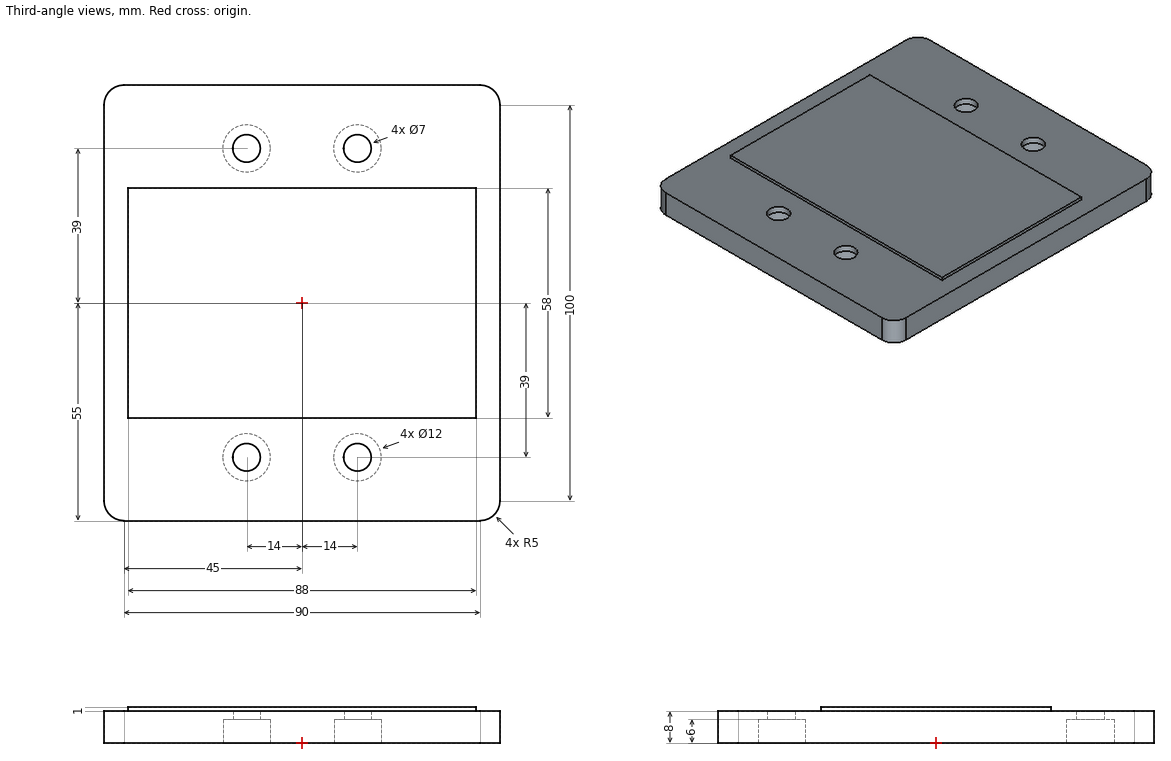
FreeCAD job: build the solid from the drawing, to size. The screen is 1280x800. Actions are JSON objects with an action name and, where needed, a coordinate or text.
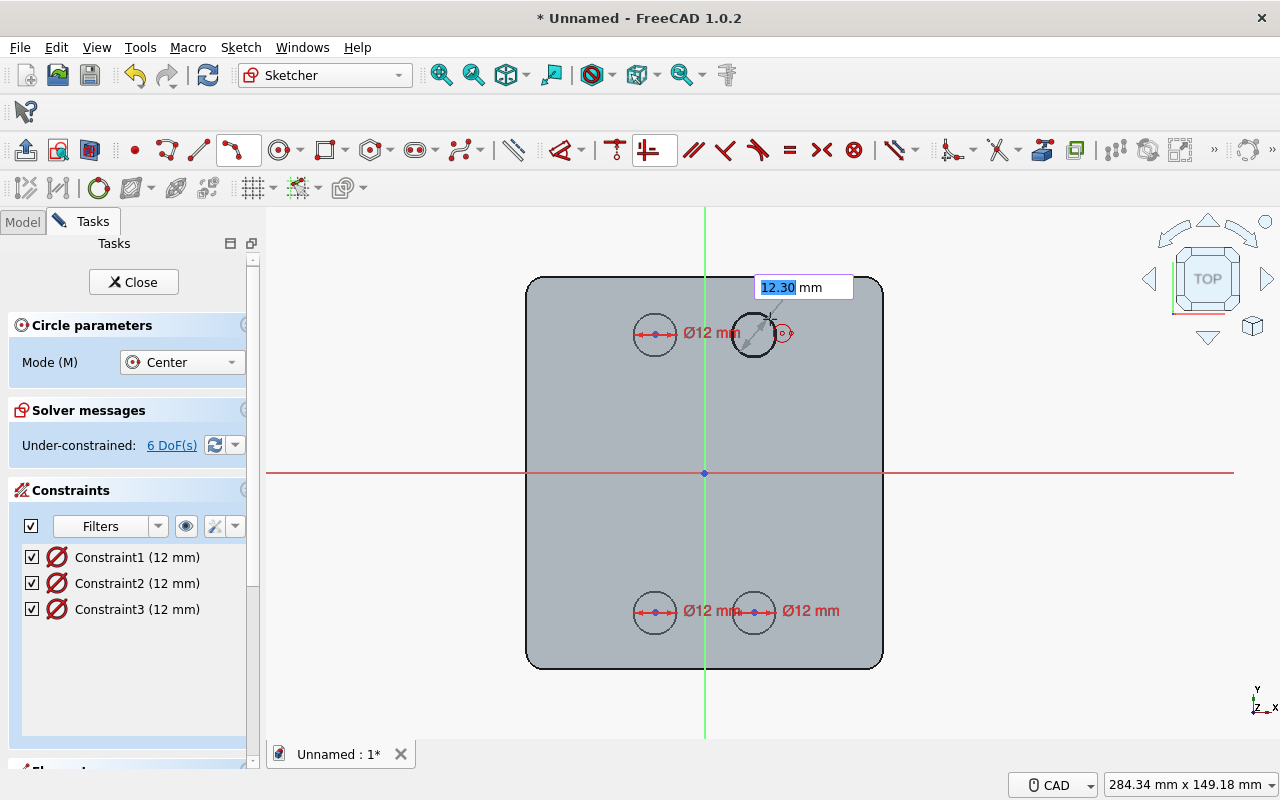
{"action": "type", "text": "12"}
{"action": "key", "text": "Return"}
{"action": "key", "text": "Escape"}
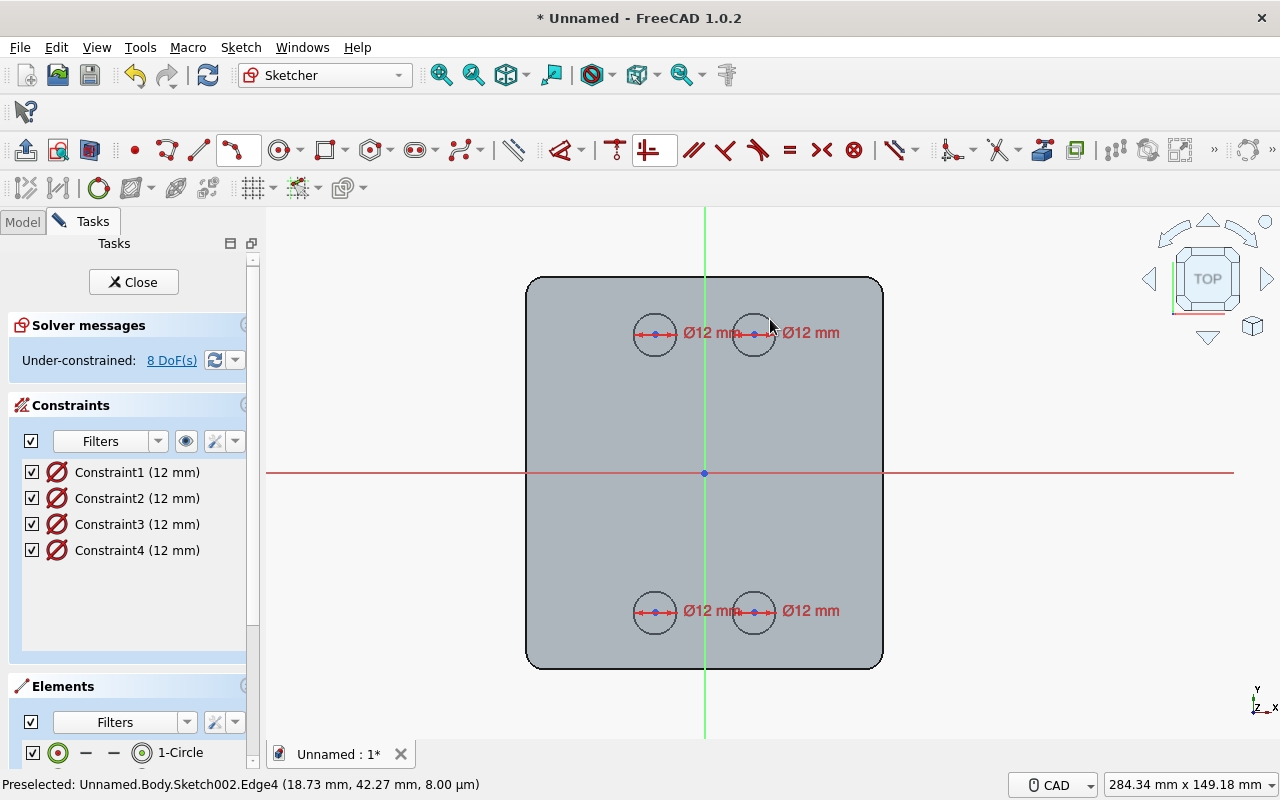
{"action": "left_click", "coordinate": [754, 613]}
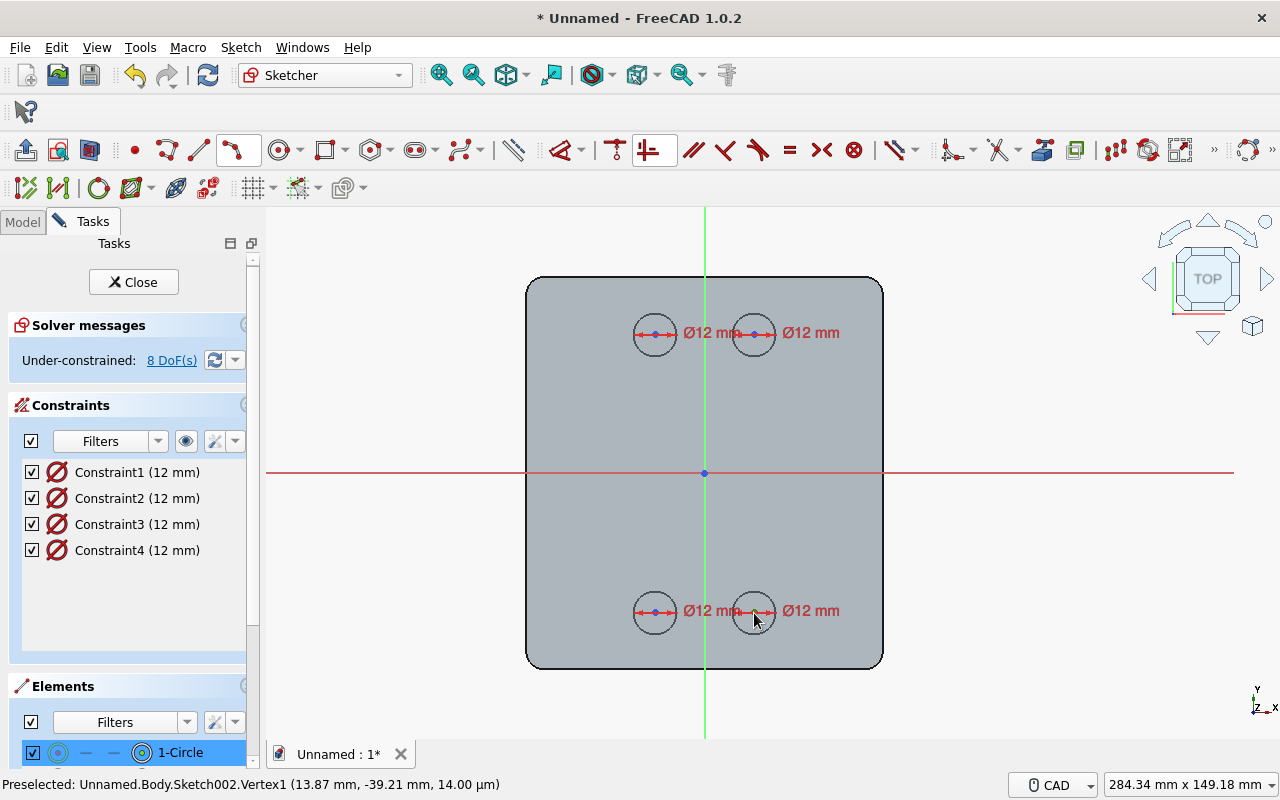
{"action": "left_click", "coordinate": [655, 613]}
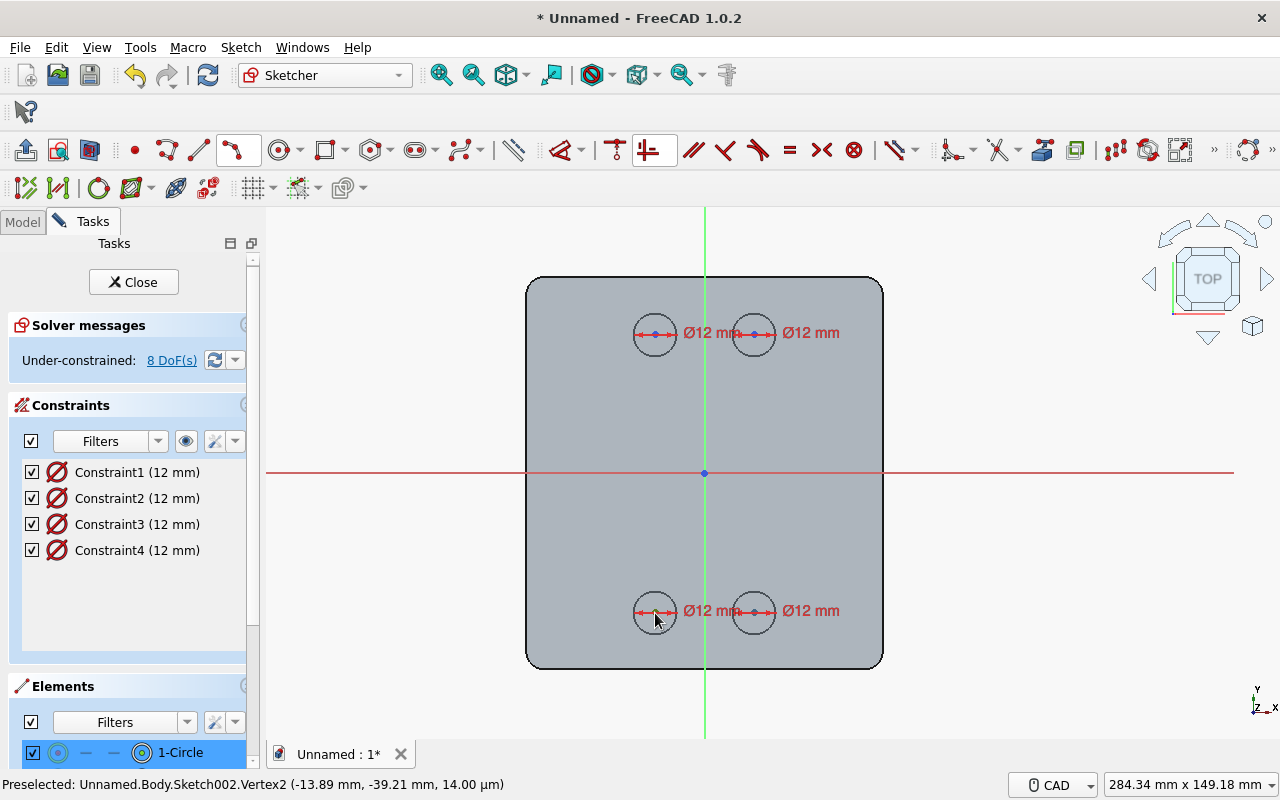
{"action": "key", "text": "h"}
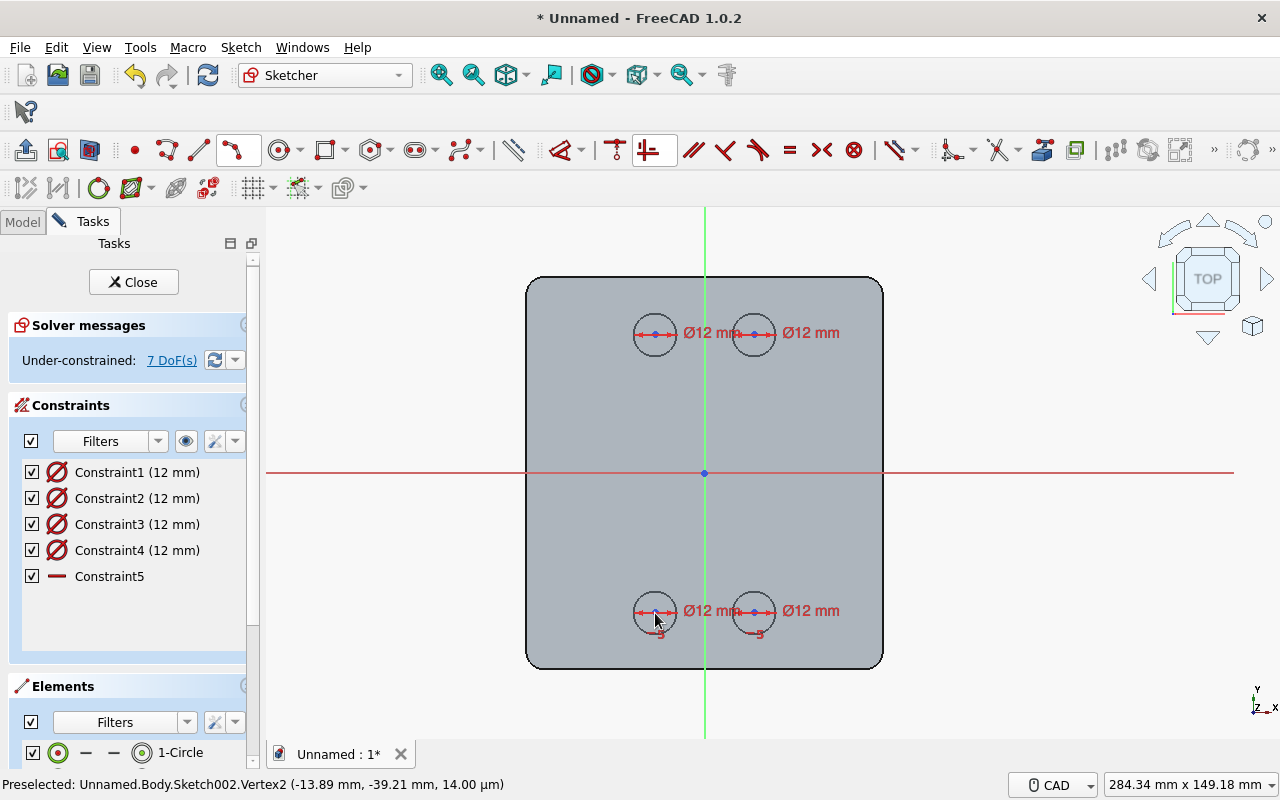
{"action": "left_click", "coordinate": [655, 613]}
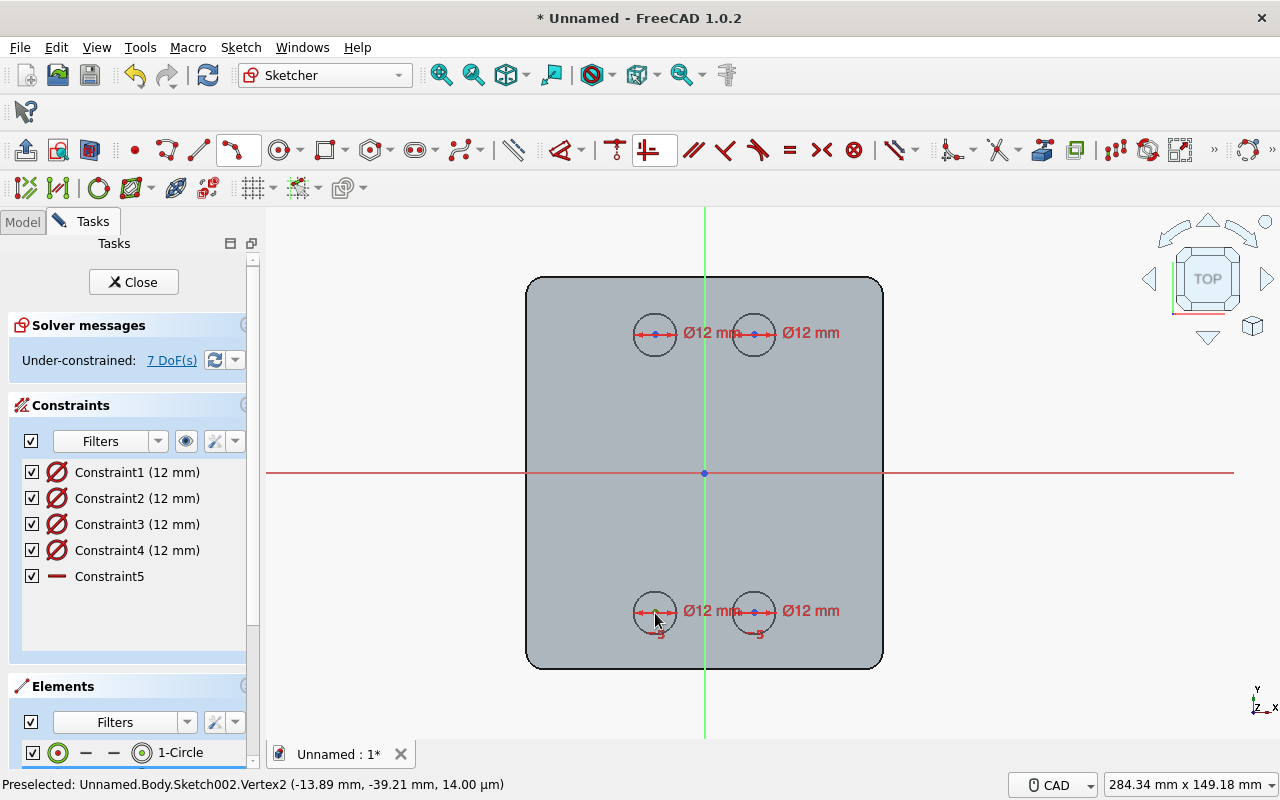
{"action": "left_click", "coordinate": [655, 335]}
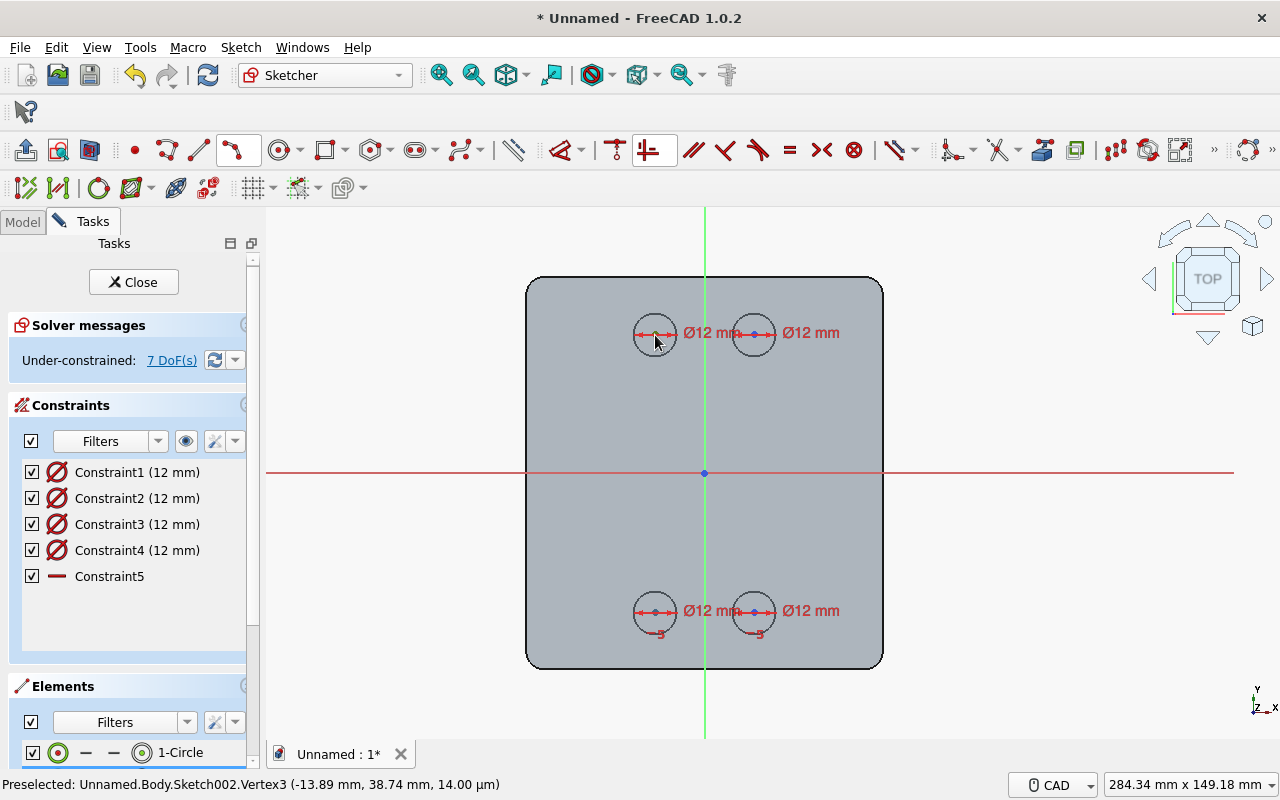
{"action": "key", "text": "v"}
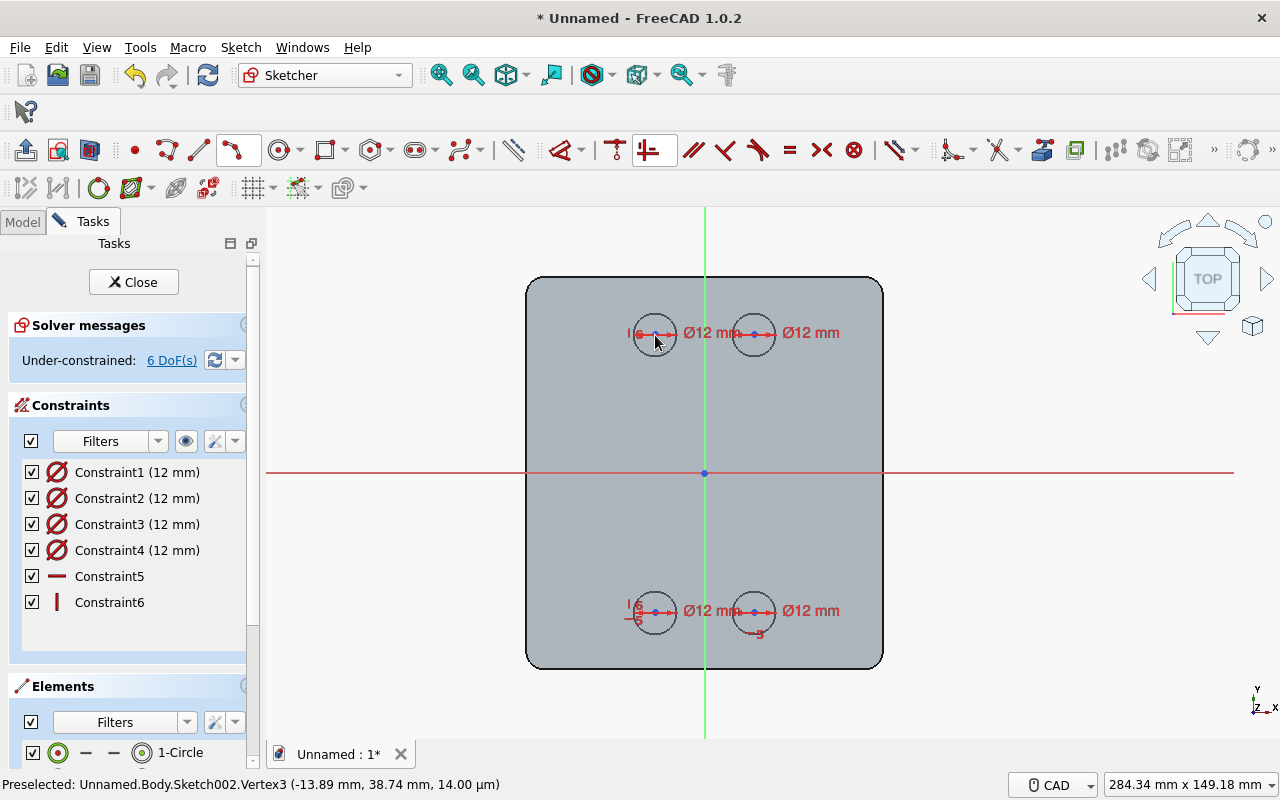
{"action": "left_click", "coordinate": [754, 613]}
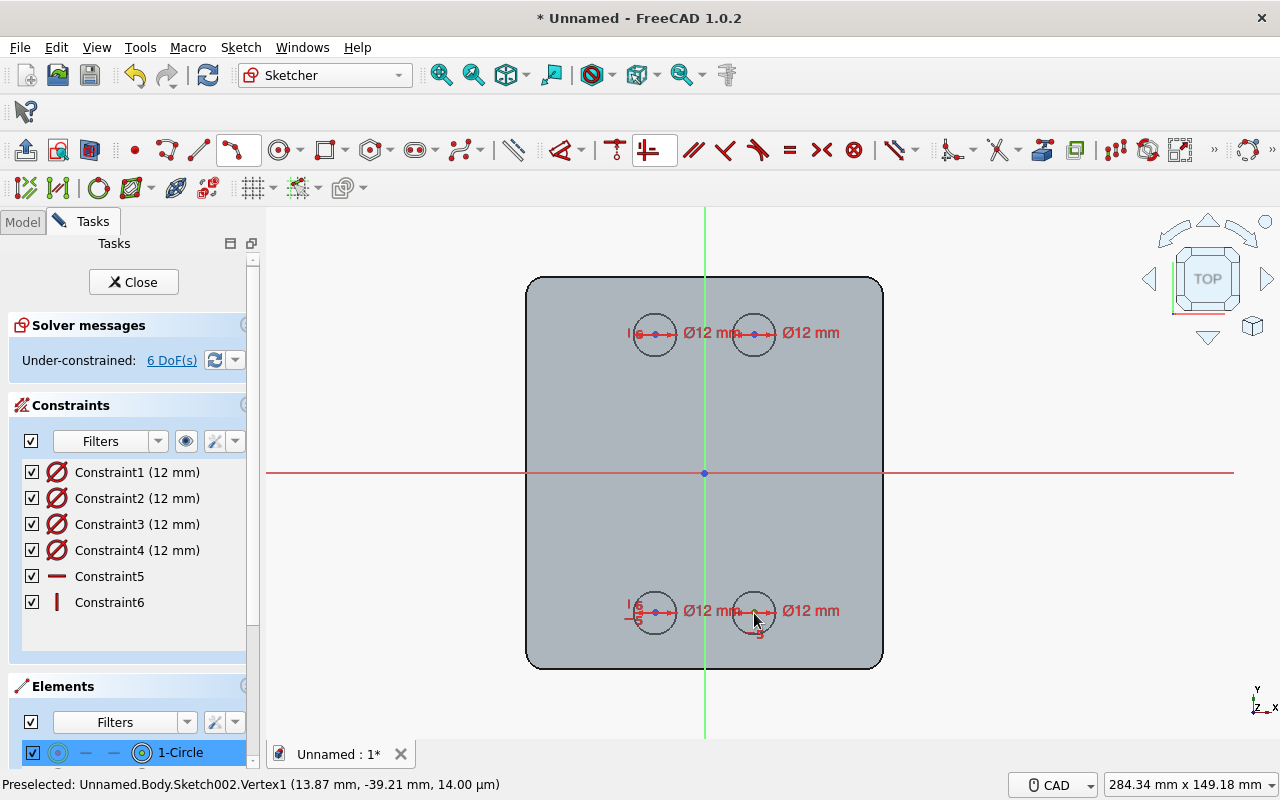
{"action": "left_click", "coordinate": [754, 335]}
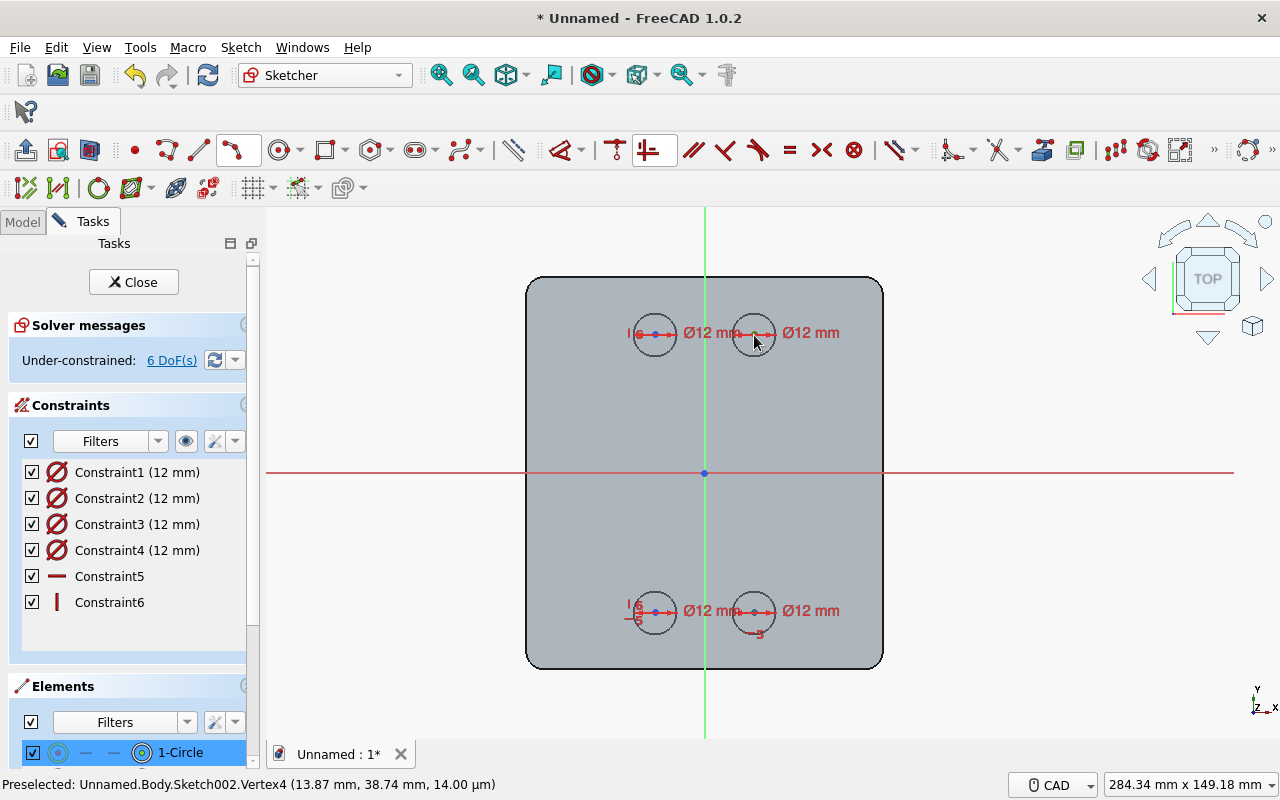
{"action": "key", "text": "v"}